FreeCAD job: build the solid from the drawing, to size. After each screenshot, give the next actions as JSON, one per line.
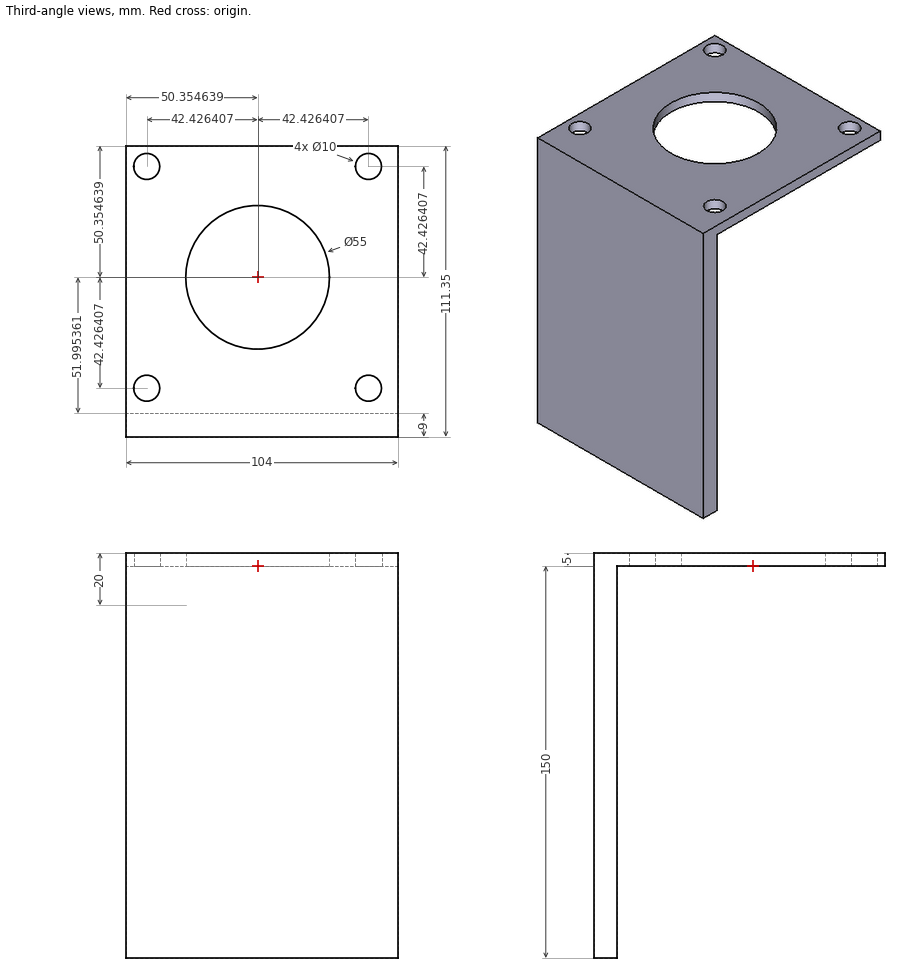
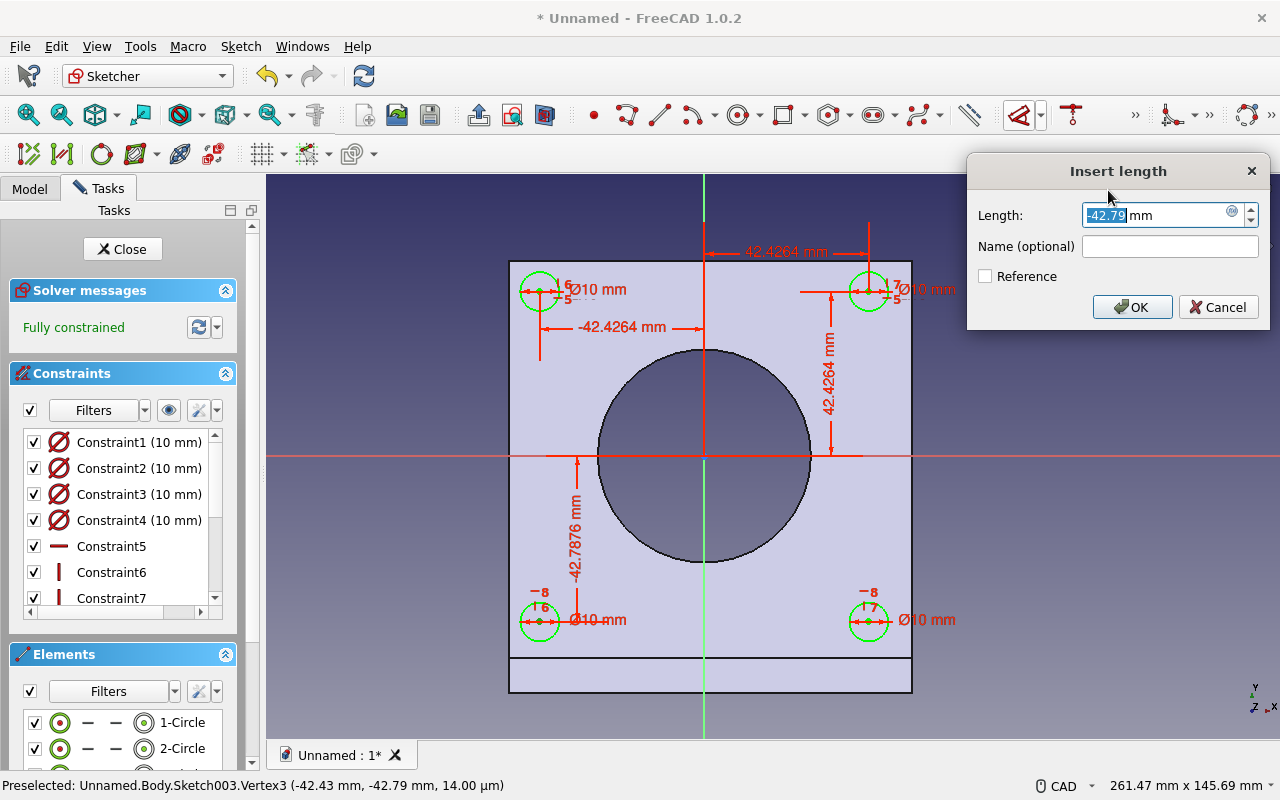
{"action": "type", "text": "-42.426407"}
{"action": "key", "text": "Return"}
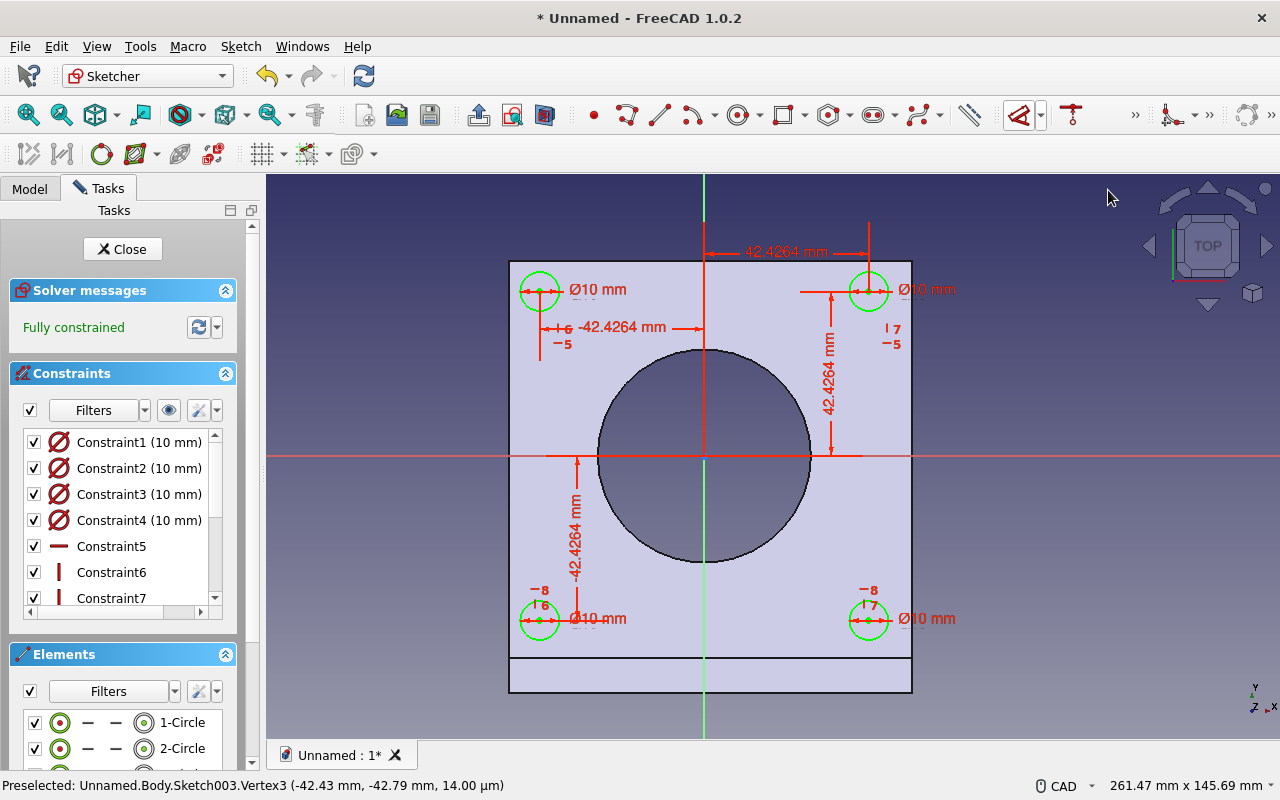
{"action": "left_click", "coordinate": [123, 249]}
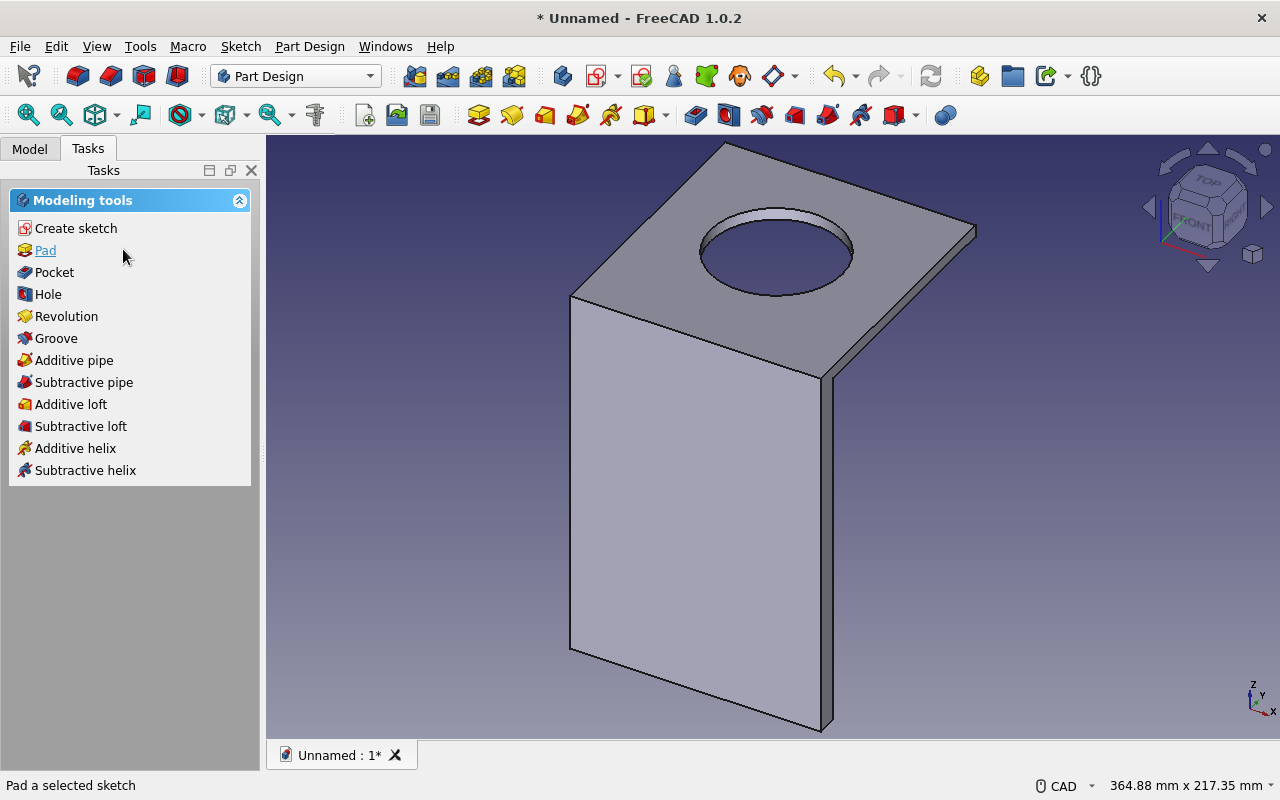
{"action": "left_click", "coordinate": [696, 116]}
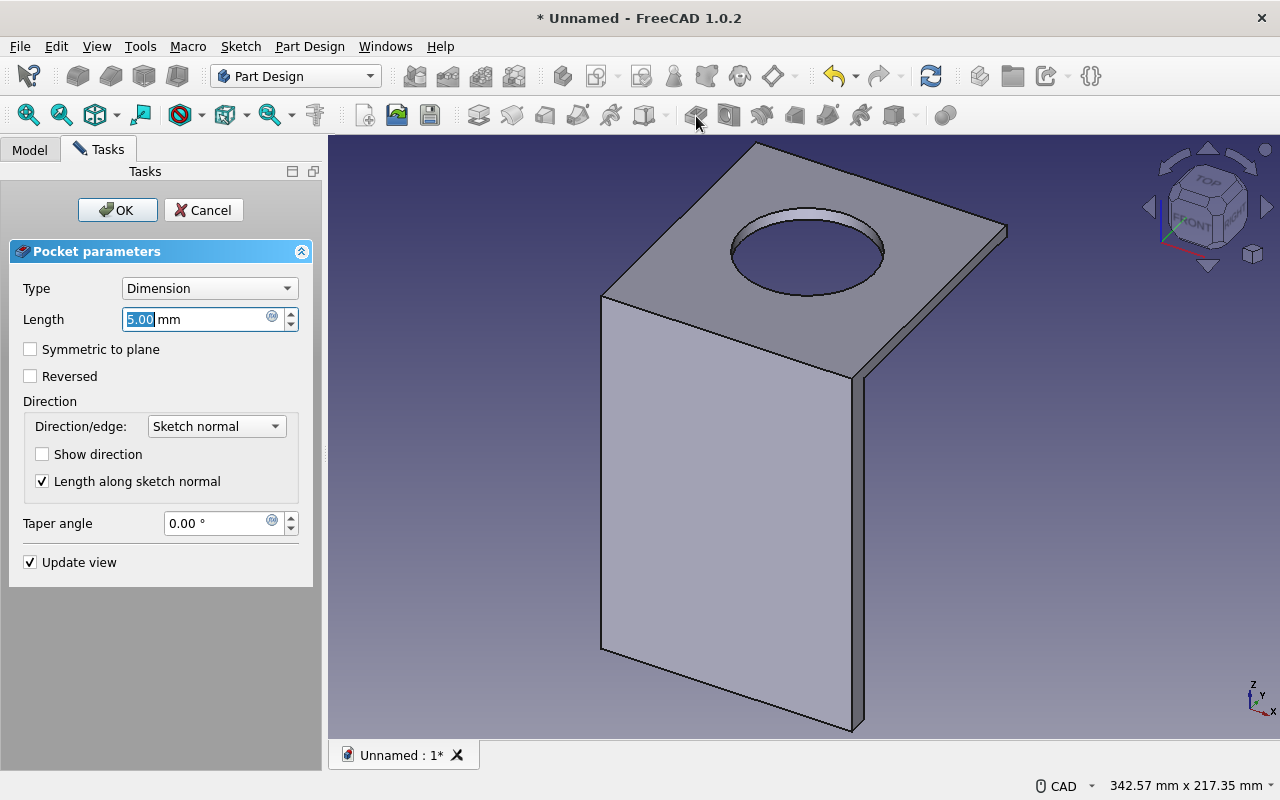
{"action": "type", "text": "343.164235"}
{"action": "key", "text": "Tab"}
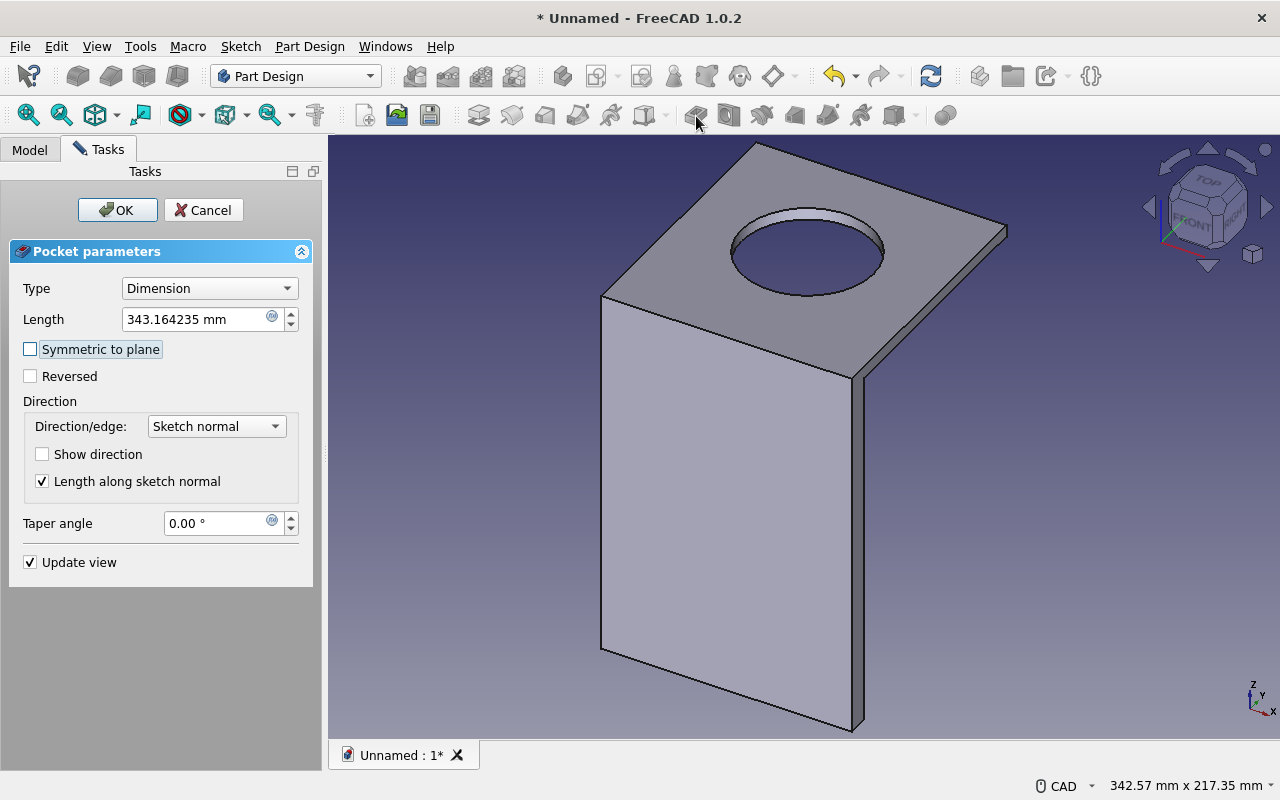
{"action": "left_click", "coordinate": [31, 349]}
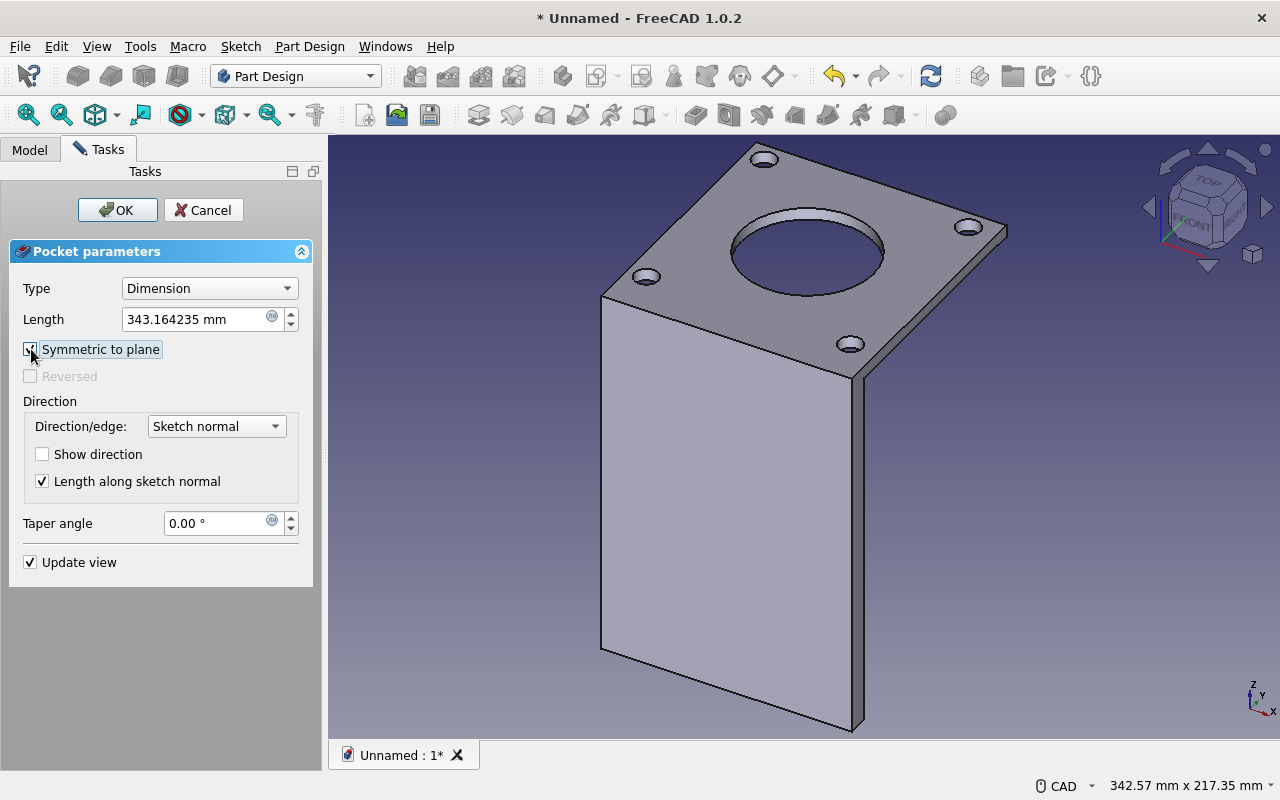
{"action": "left_click", "coordinate": [118, 210]}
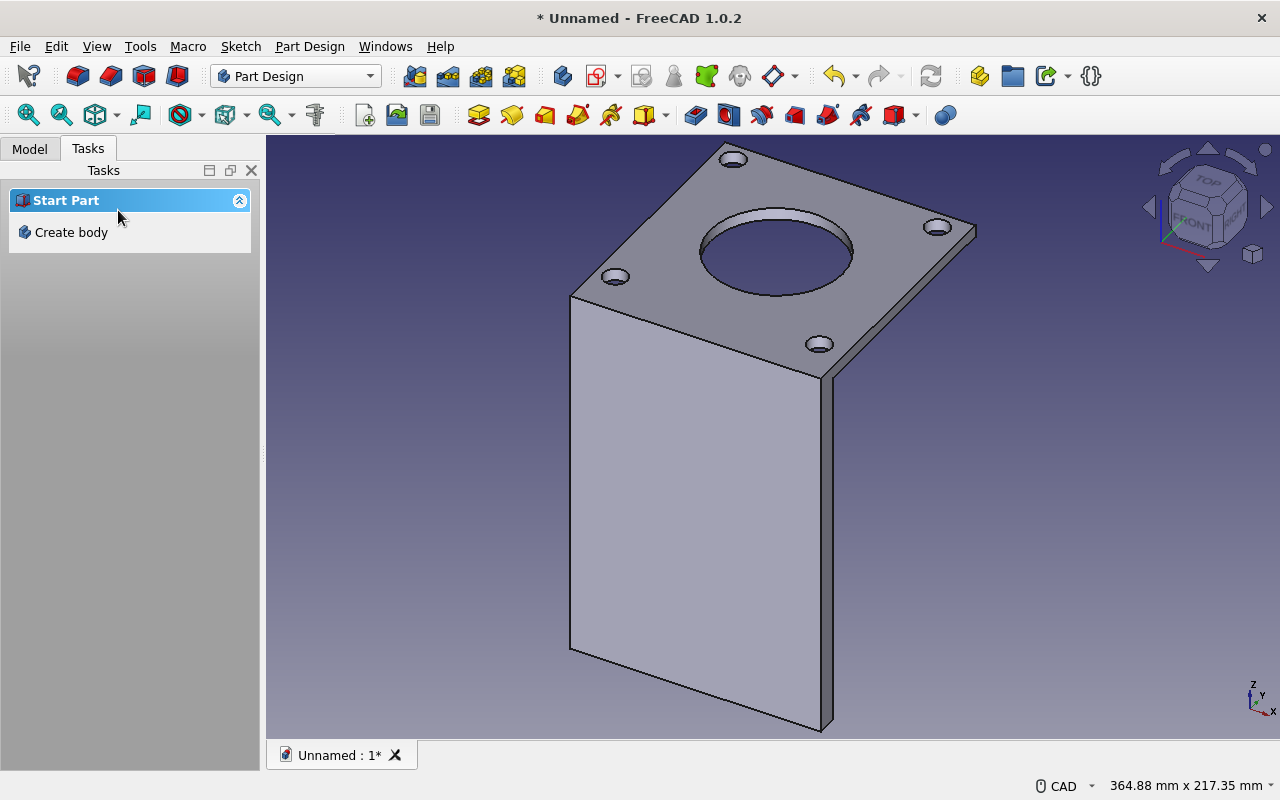
{"action": "key", "text": "0"}